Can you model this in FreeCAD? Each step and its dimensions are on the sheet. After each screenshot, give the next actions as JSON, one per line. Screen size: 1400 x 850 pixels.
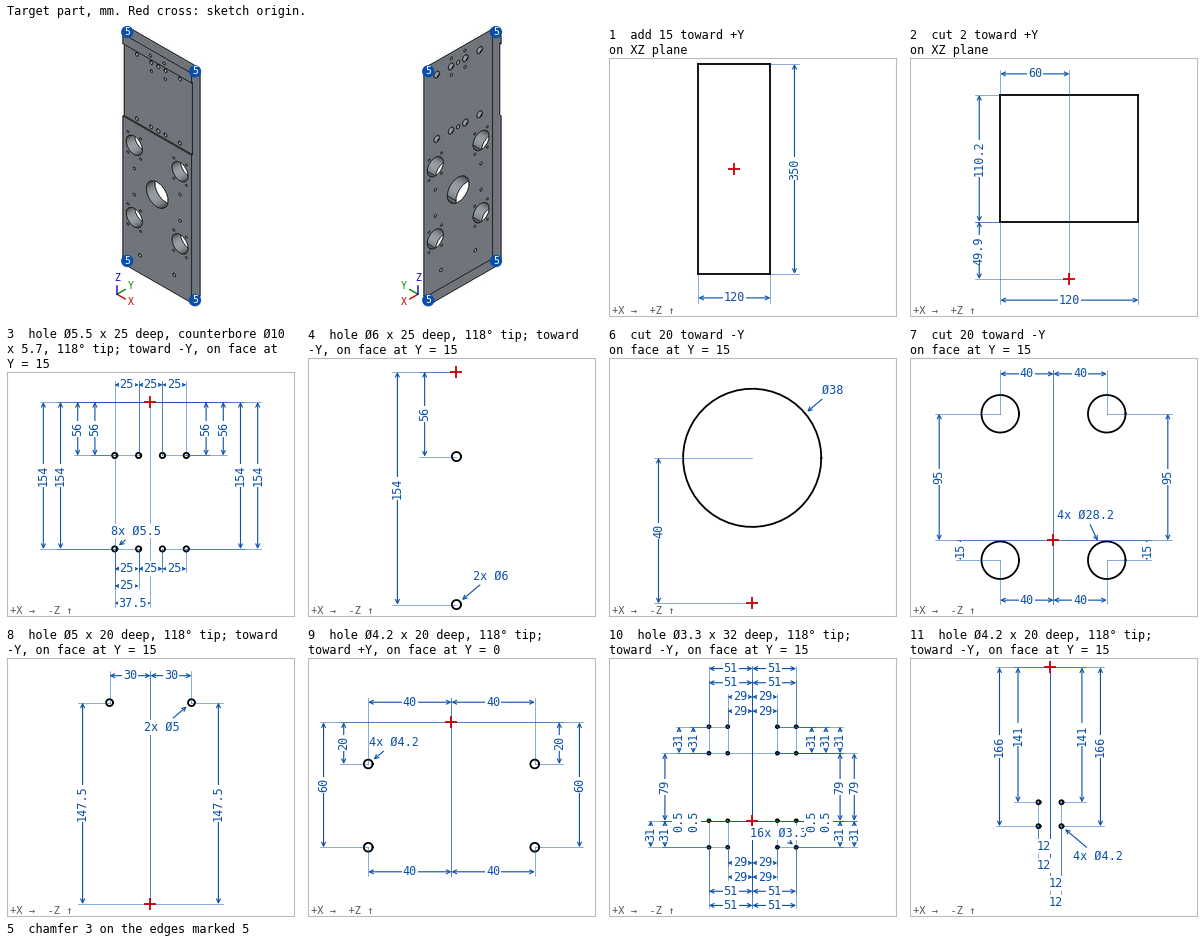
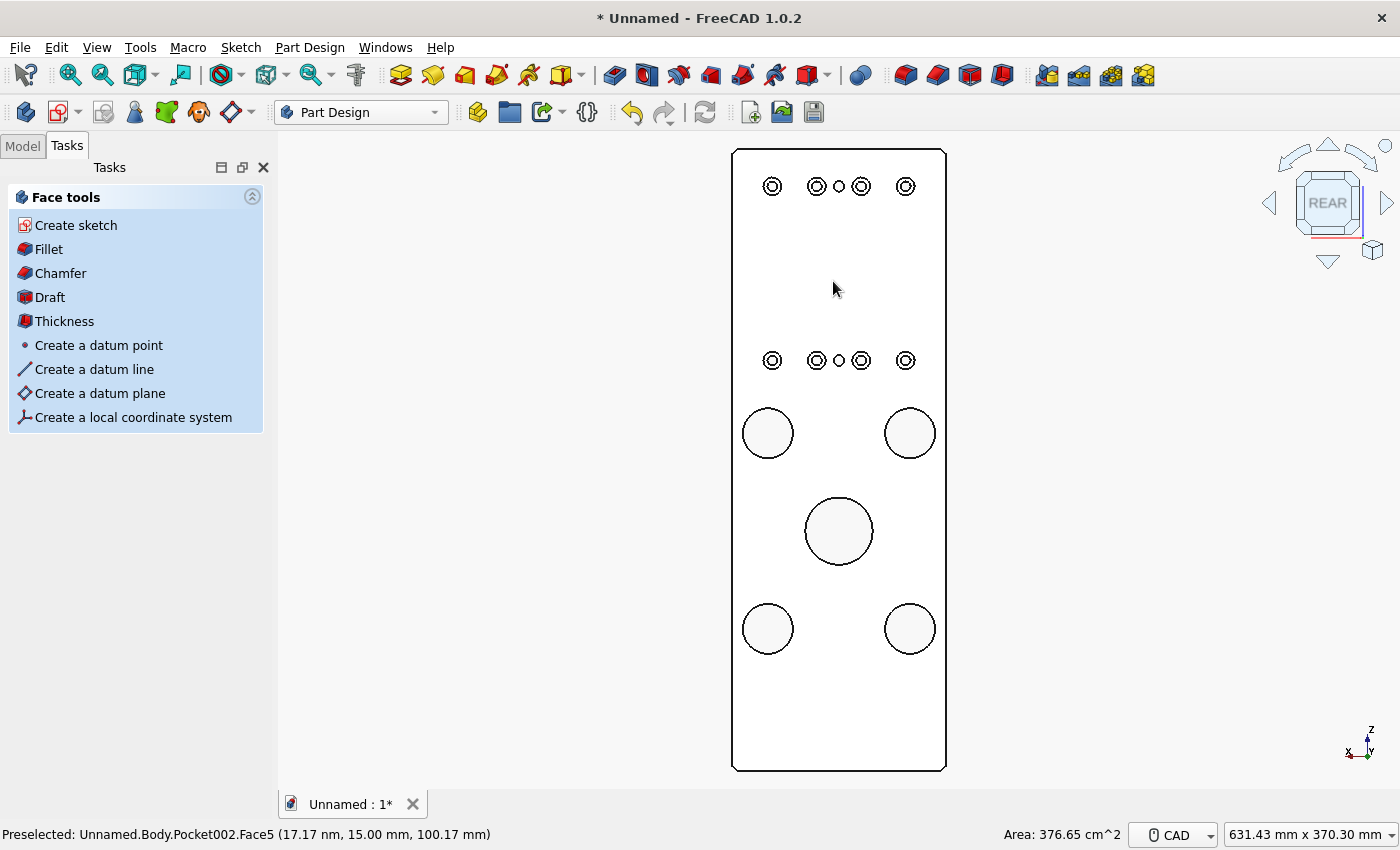
{"action": "left_click", "coordinate": [58, 112]}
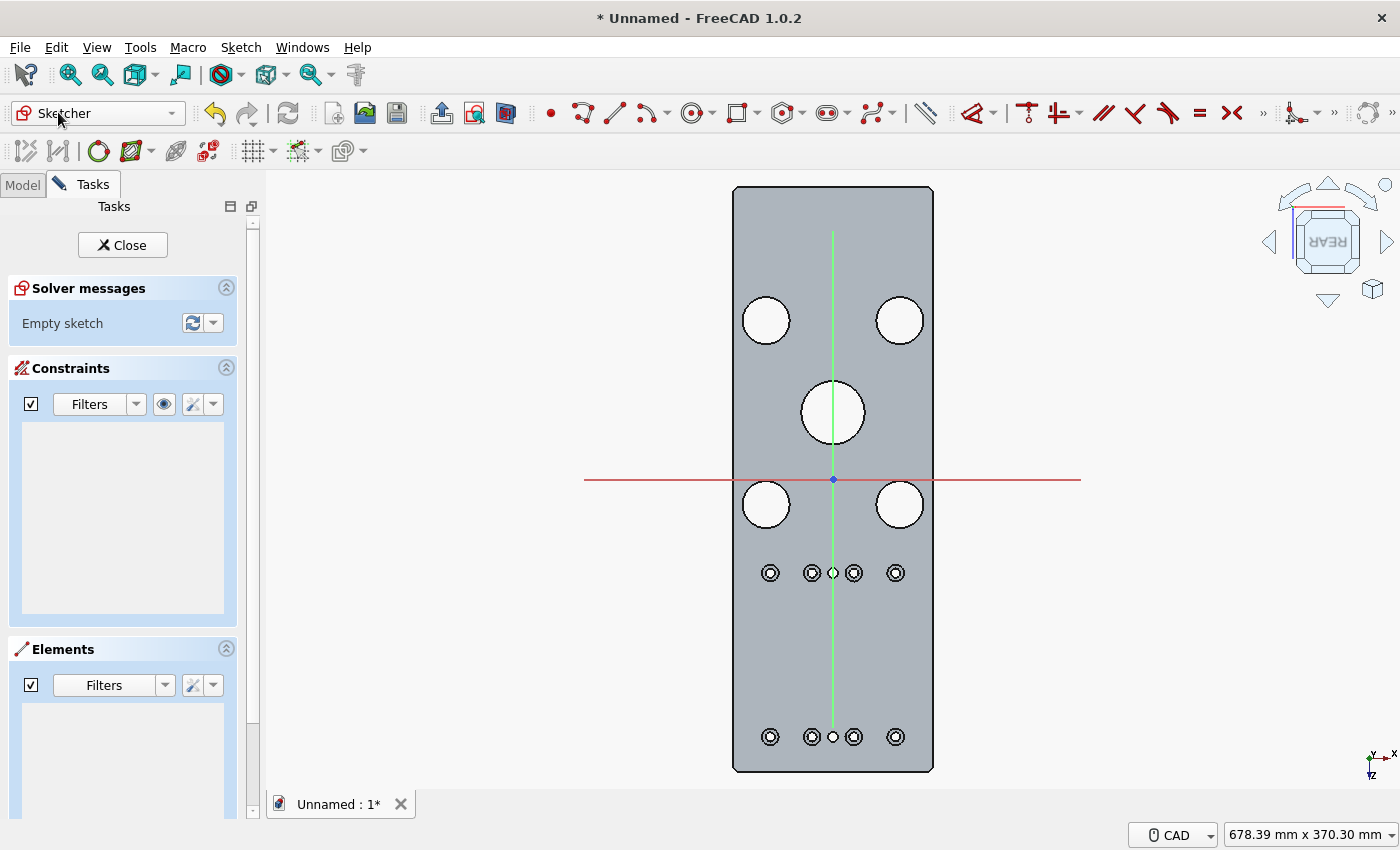
{"action": "scroll", "coordinate": [972, 198], "scroll_direction": "up", "scroll_amount": 2}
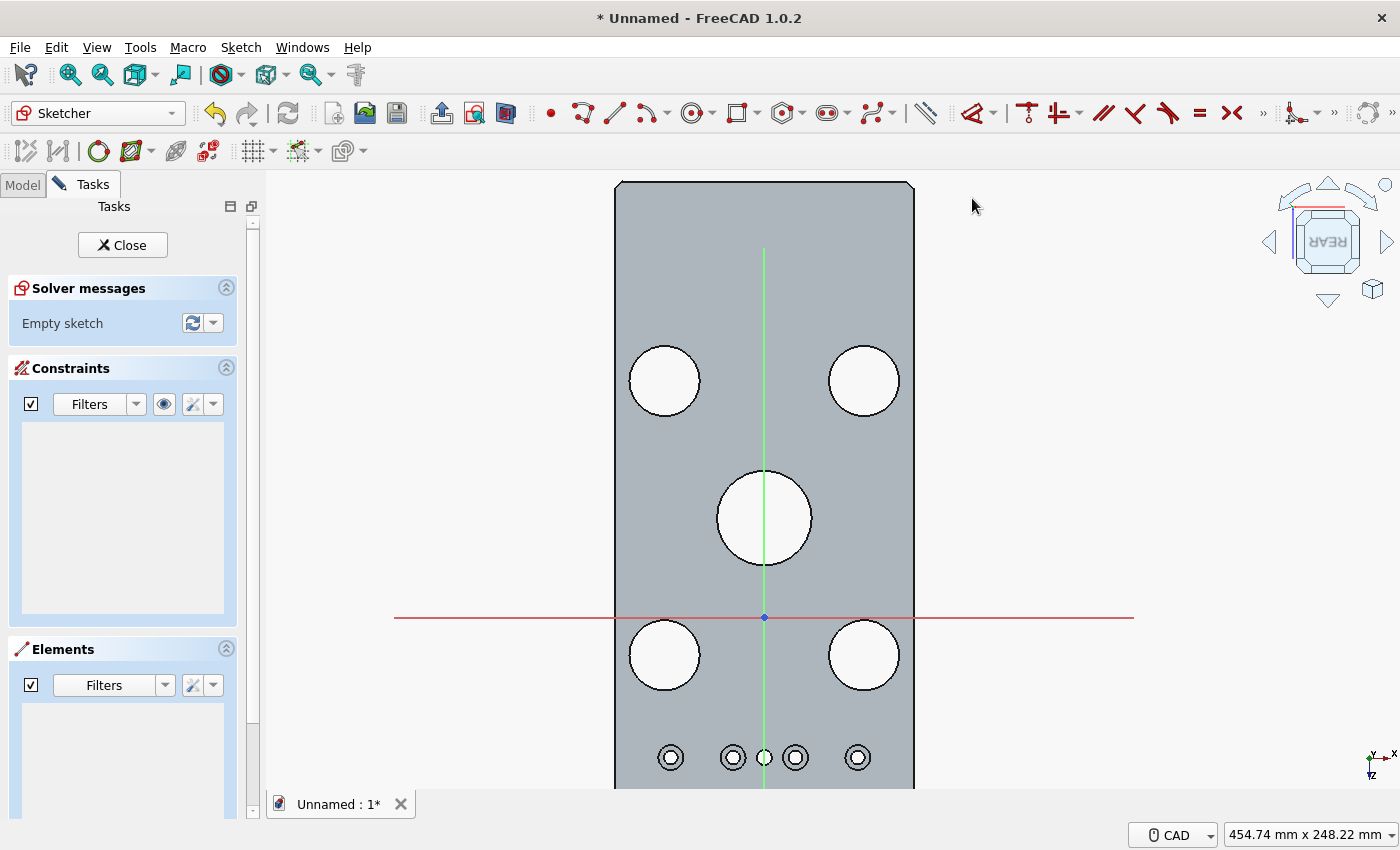
{"action": "left_click", "coordinate": [692, 114]}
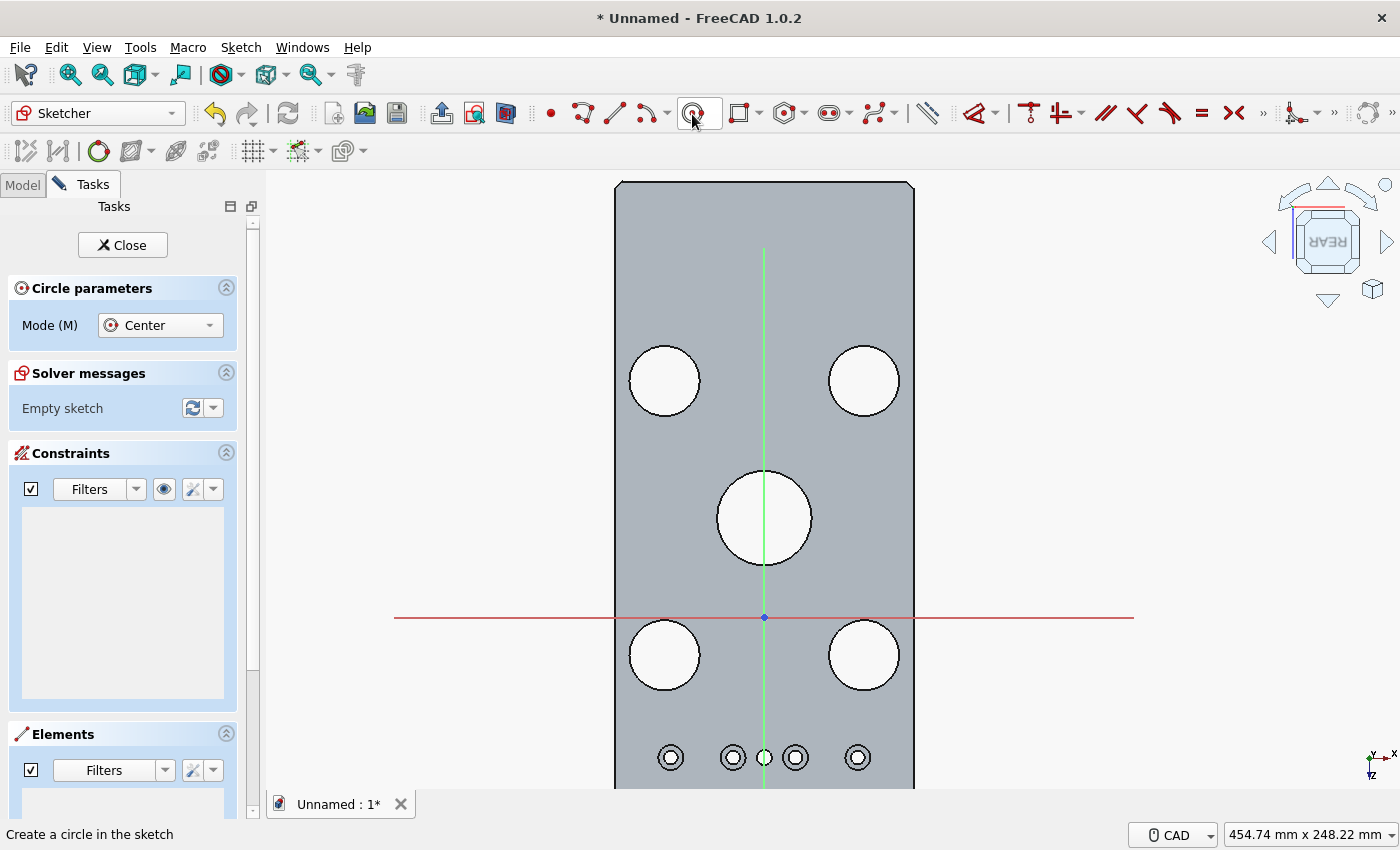
{"action": "scroll", "coordinate": [839, 250], "scroll_direction": "up", "scroll_amount": 7}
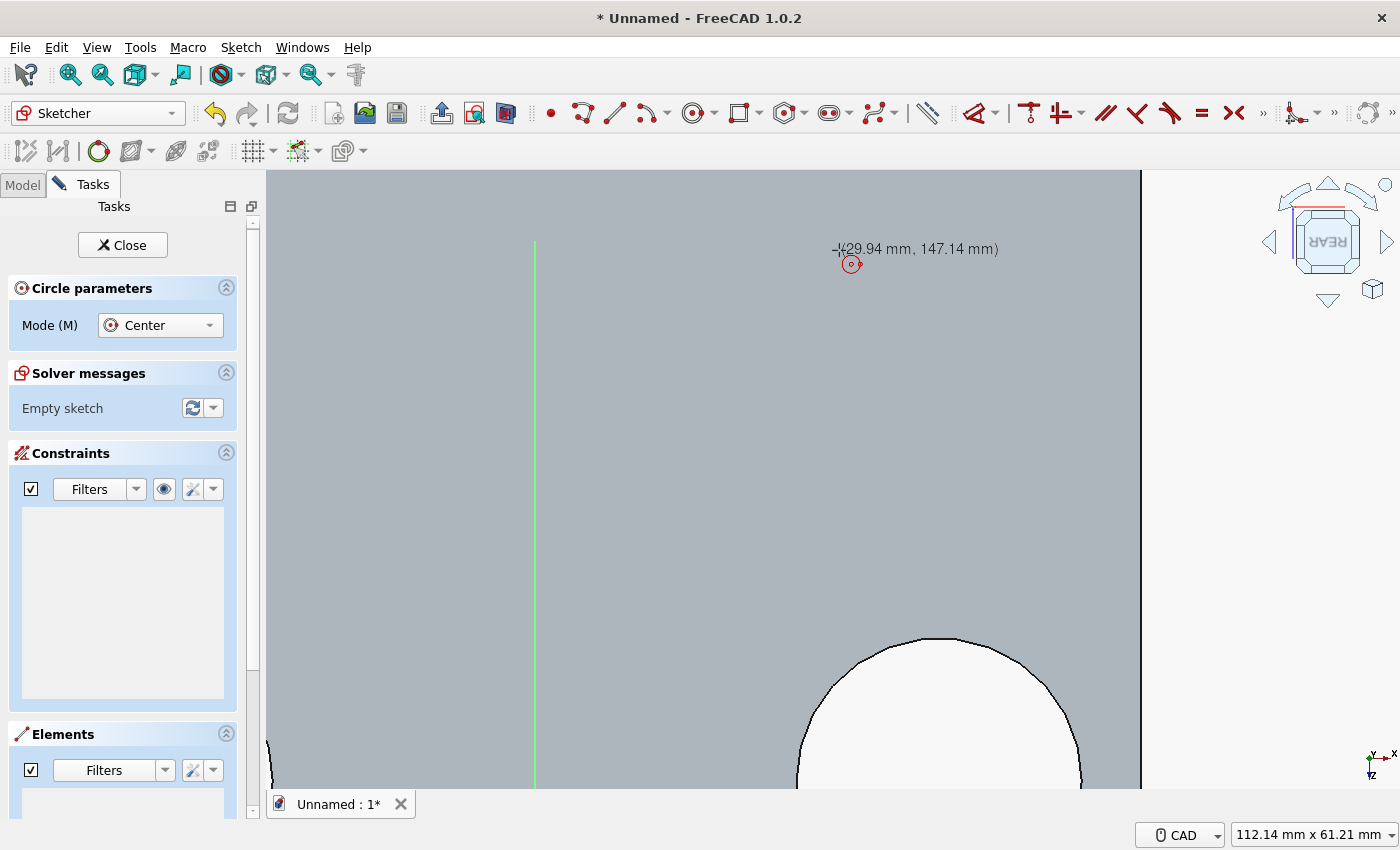
{"action": "scroll", "coordinate": [840, 315], "scroll_direction": "down", "scroll_amount": 7}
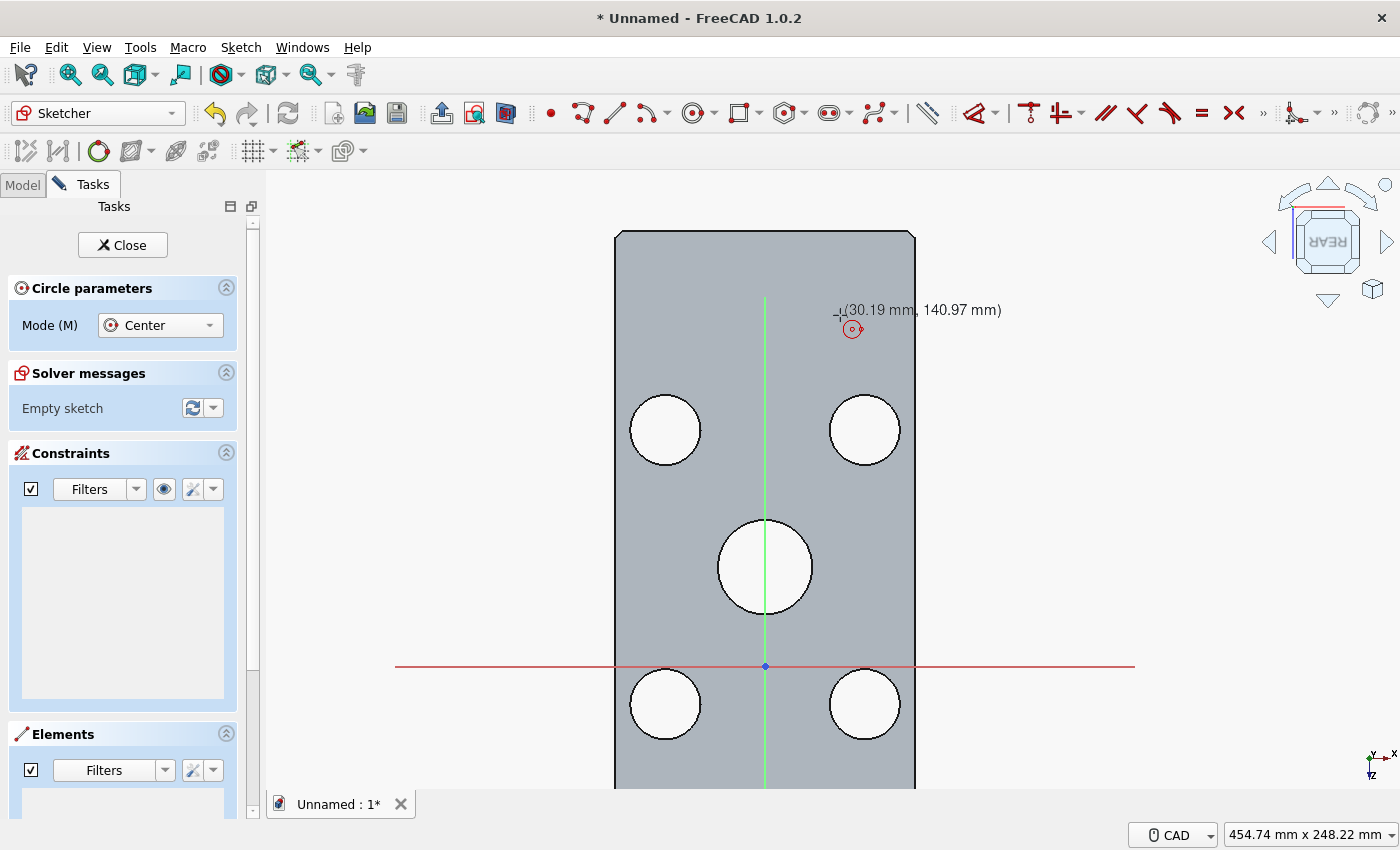
{"action": "left_click", "coordinate": [840, 299]}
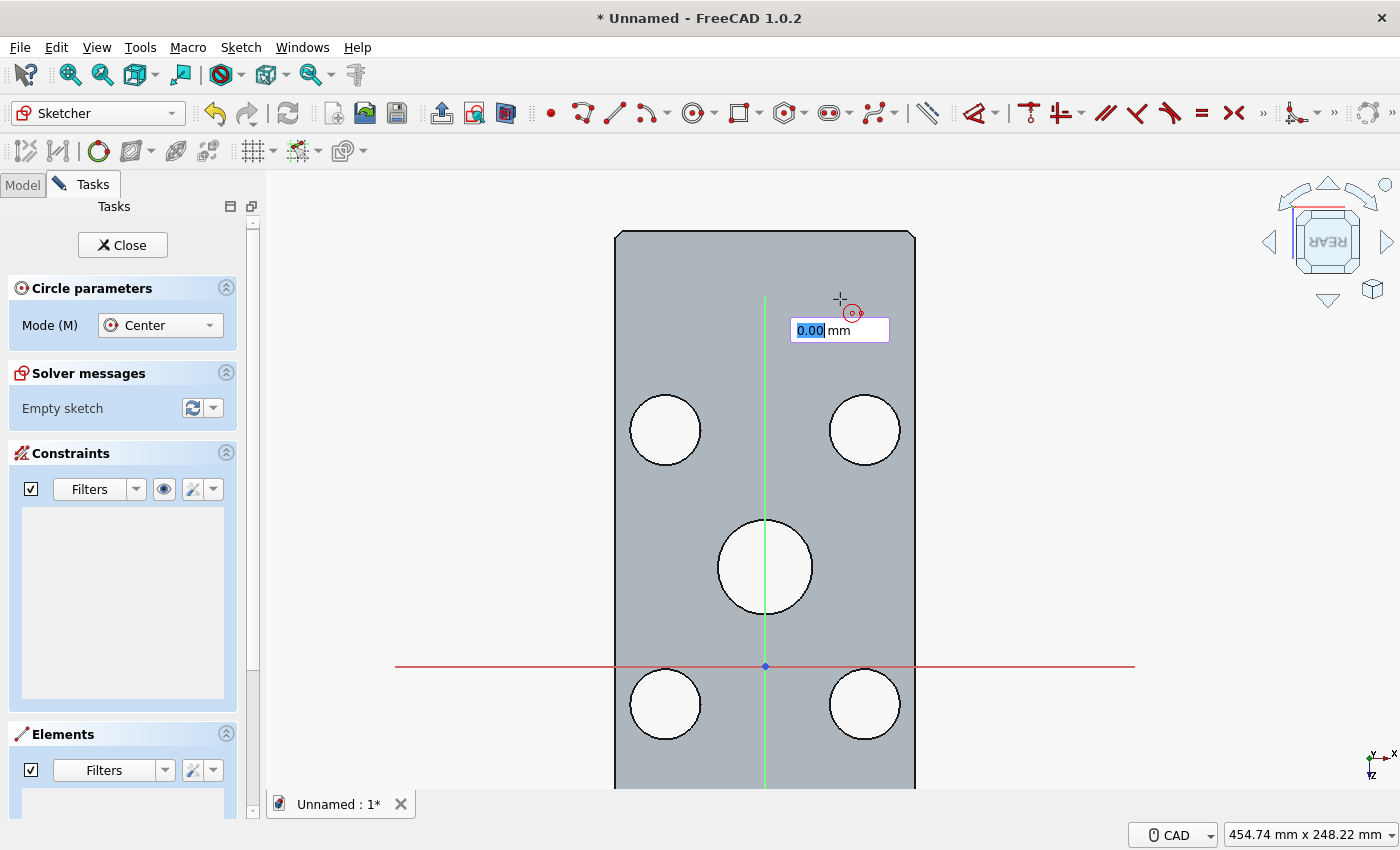
{"action": "scroll", "coordinate": [844, 295], "scroll_direction": "up", "scroll_amount": 5}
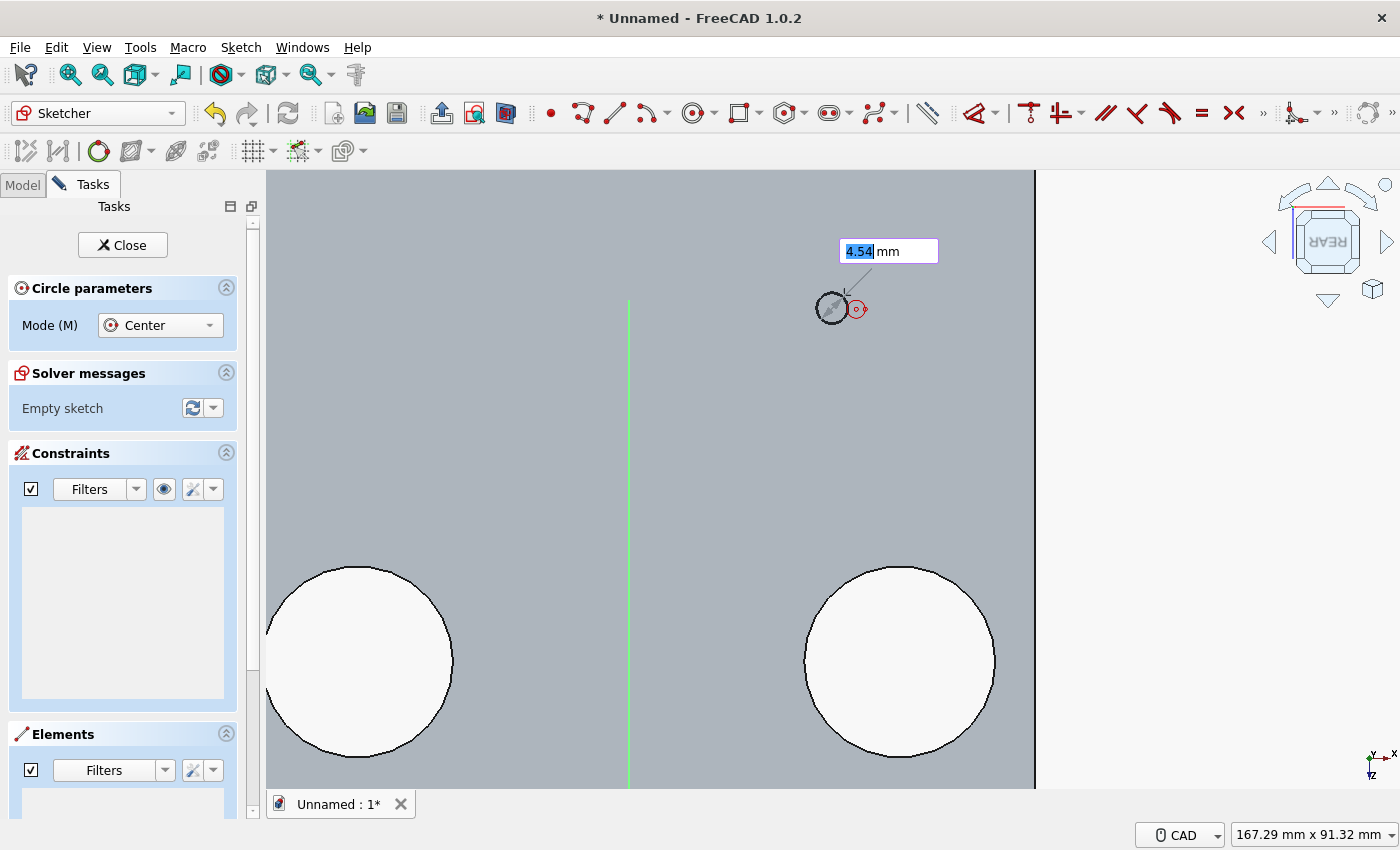
{"action": "left_click", "coordinate": [844, 294]}